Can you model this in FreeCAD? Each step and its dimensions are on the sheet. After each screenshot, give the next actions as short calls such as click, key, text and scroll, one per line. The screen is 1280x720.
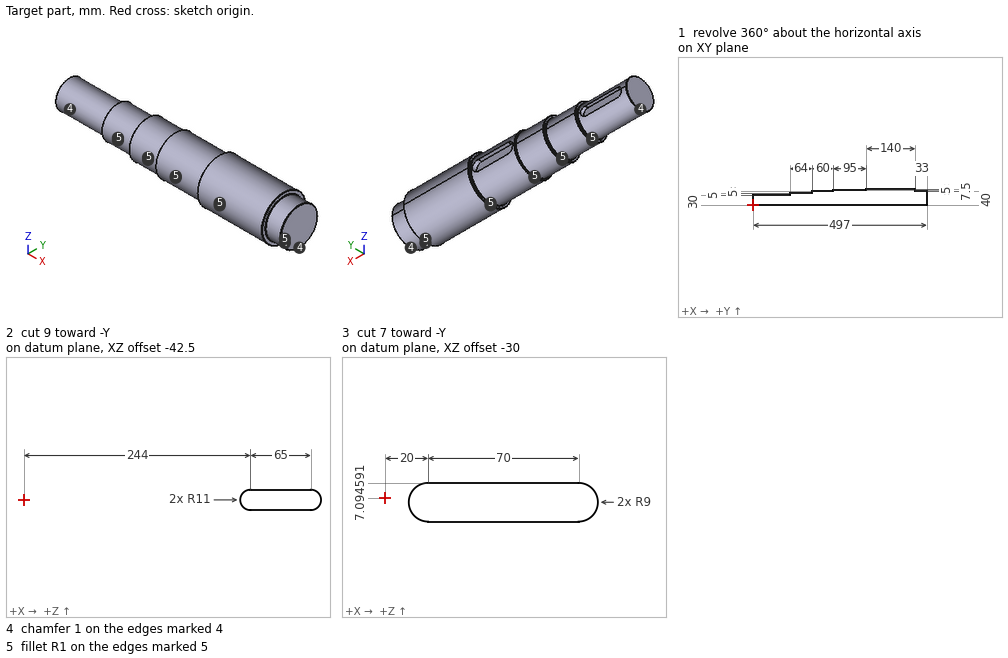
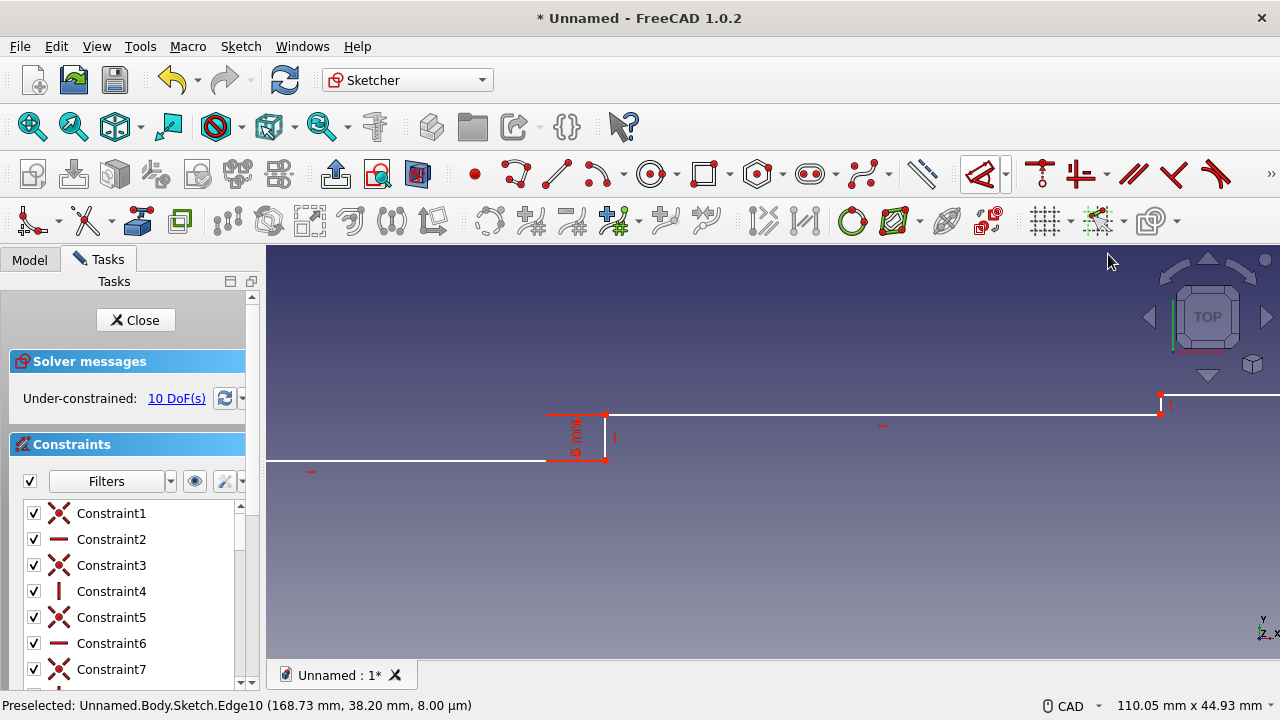
scroll(605, 435, down, 10)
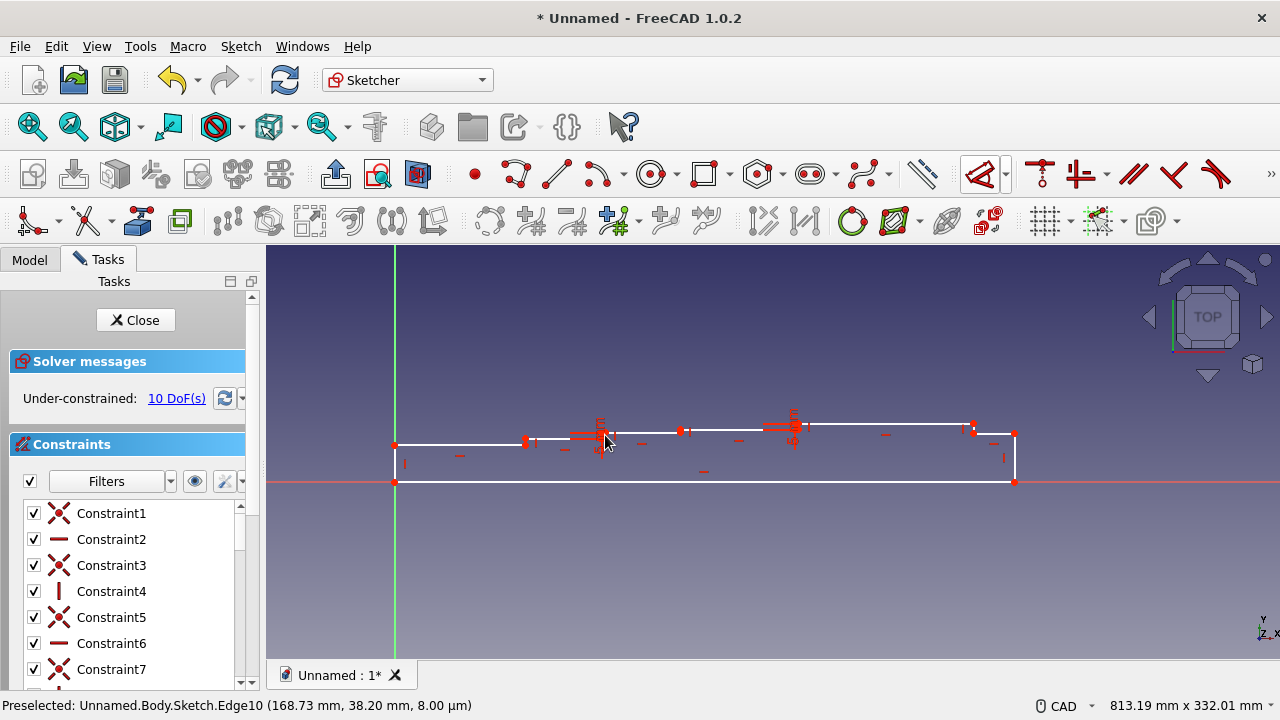
scroll(526, 441, up, 10)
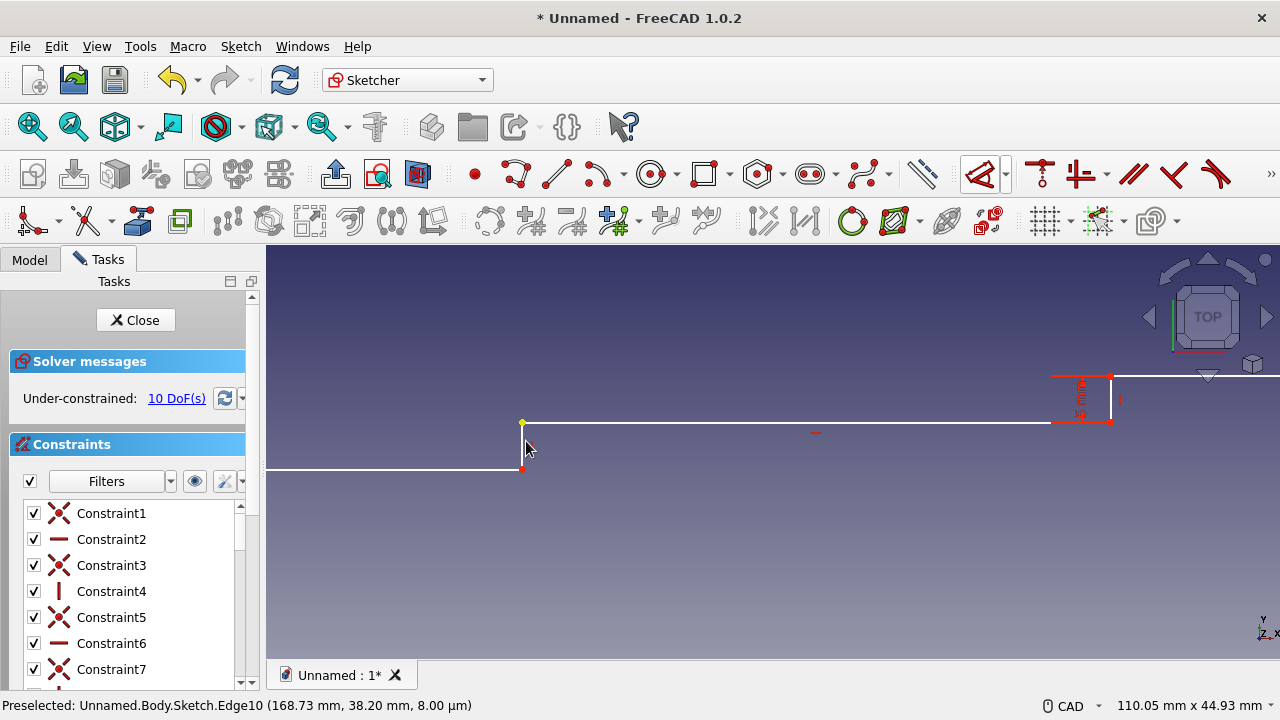
click(522, 437)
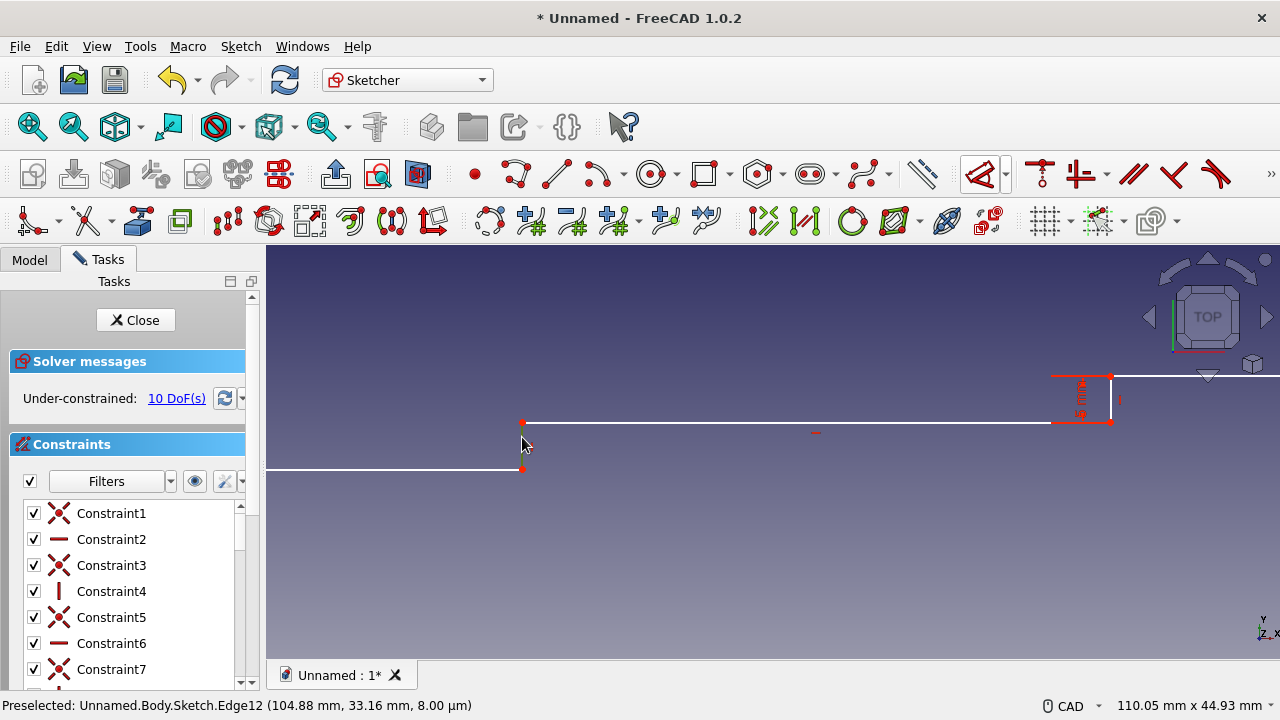
key(i)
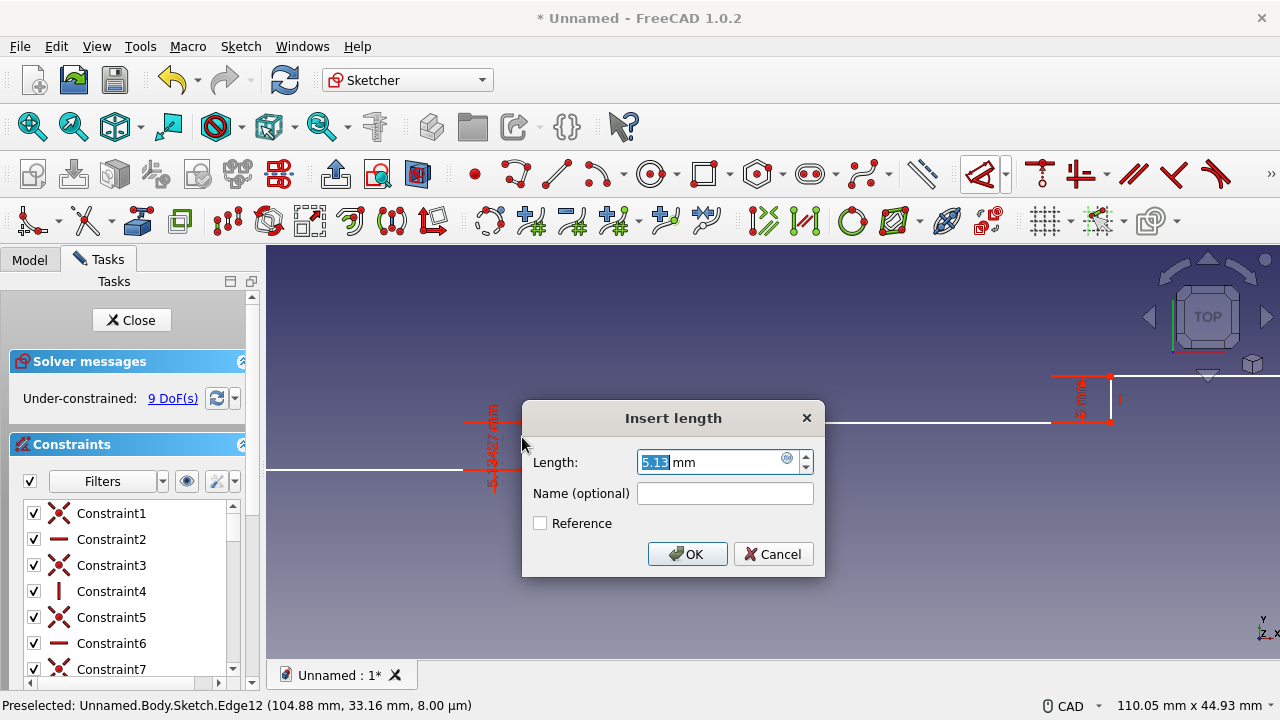
text(5)
key(Return)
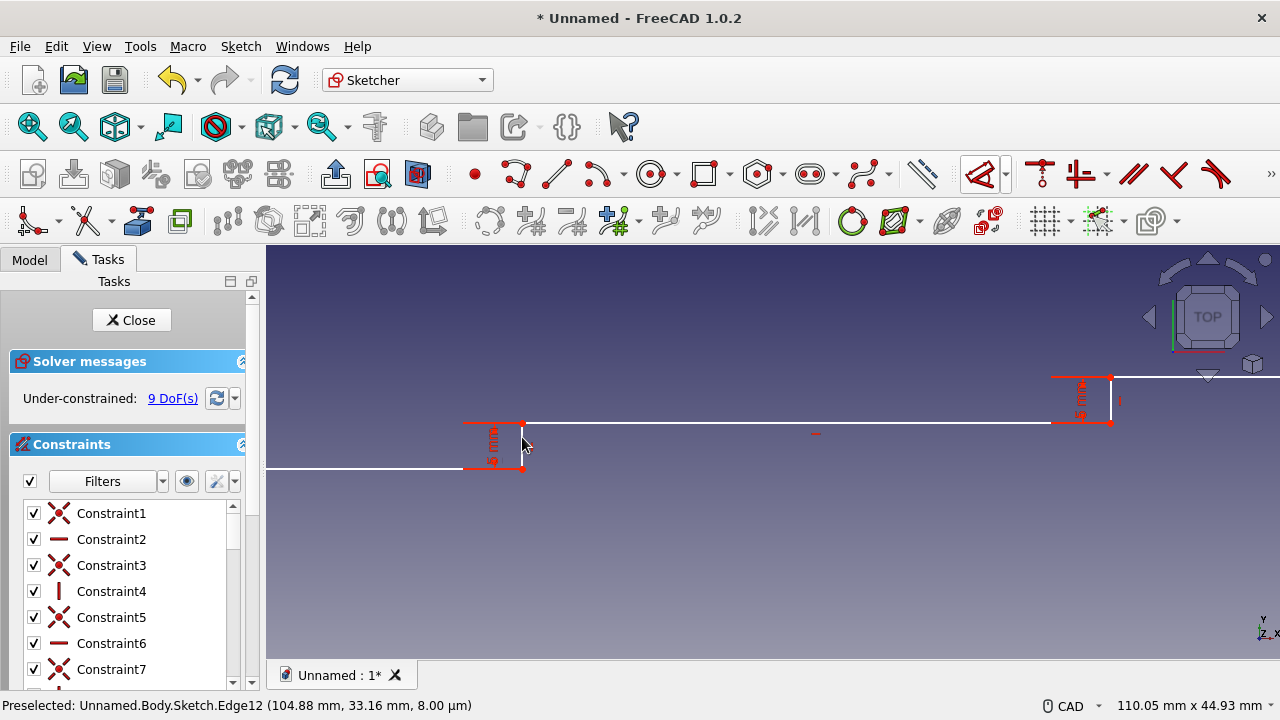
scroll(526, 441, down, 10)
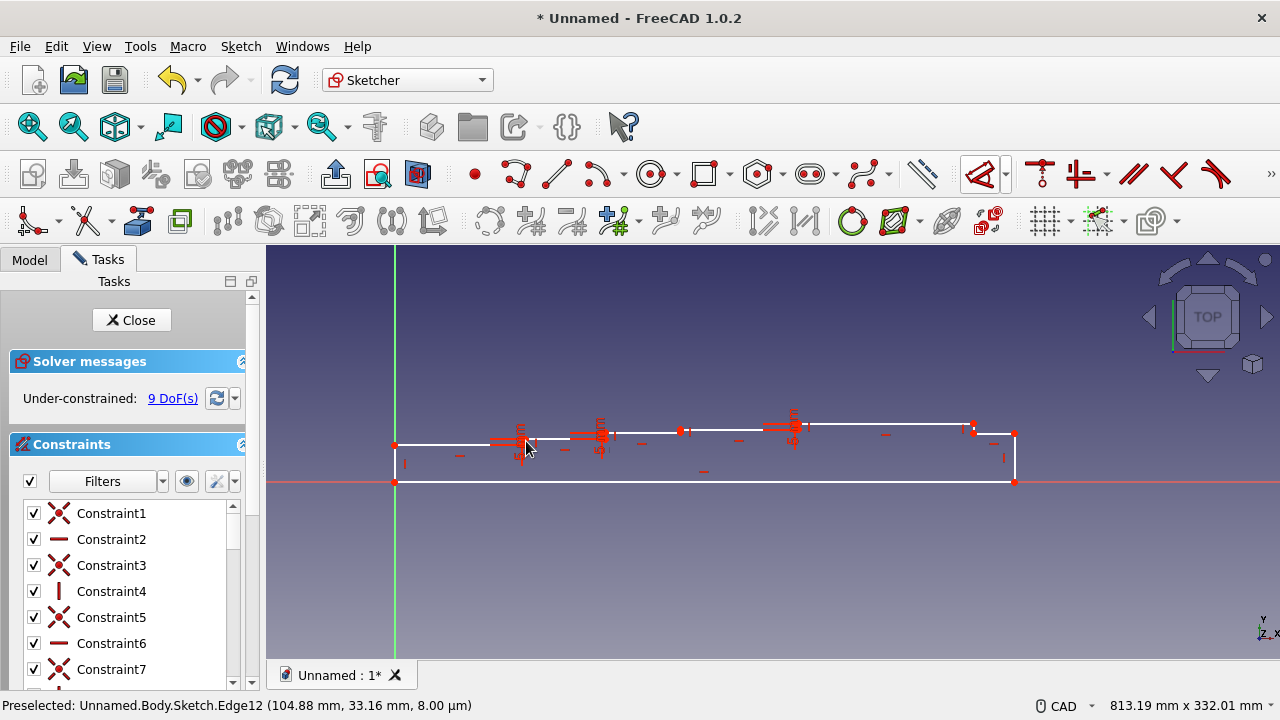
click(1015, 468)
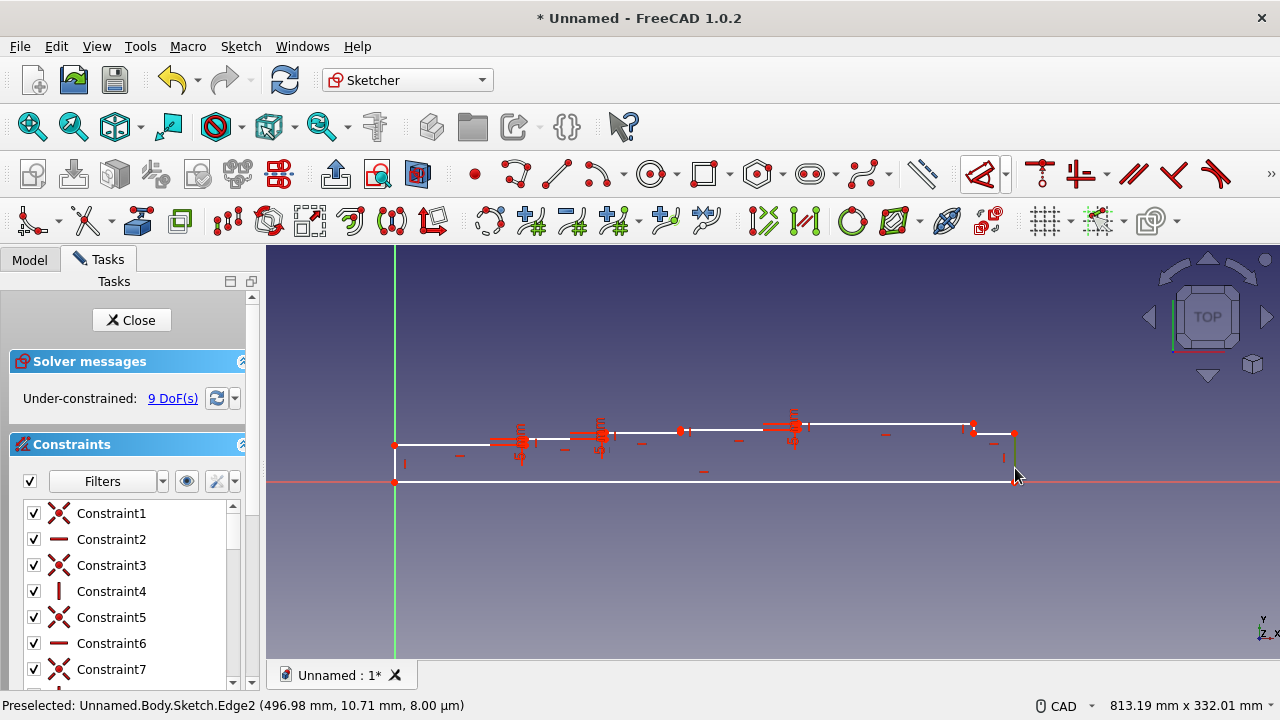
key(i)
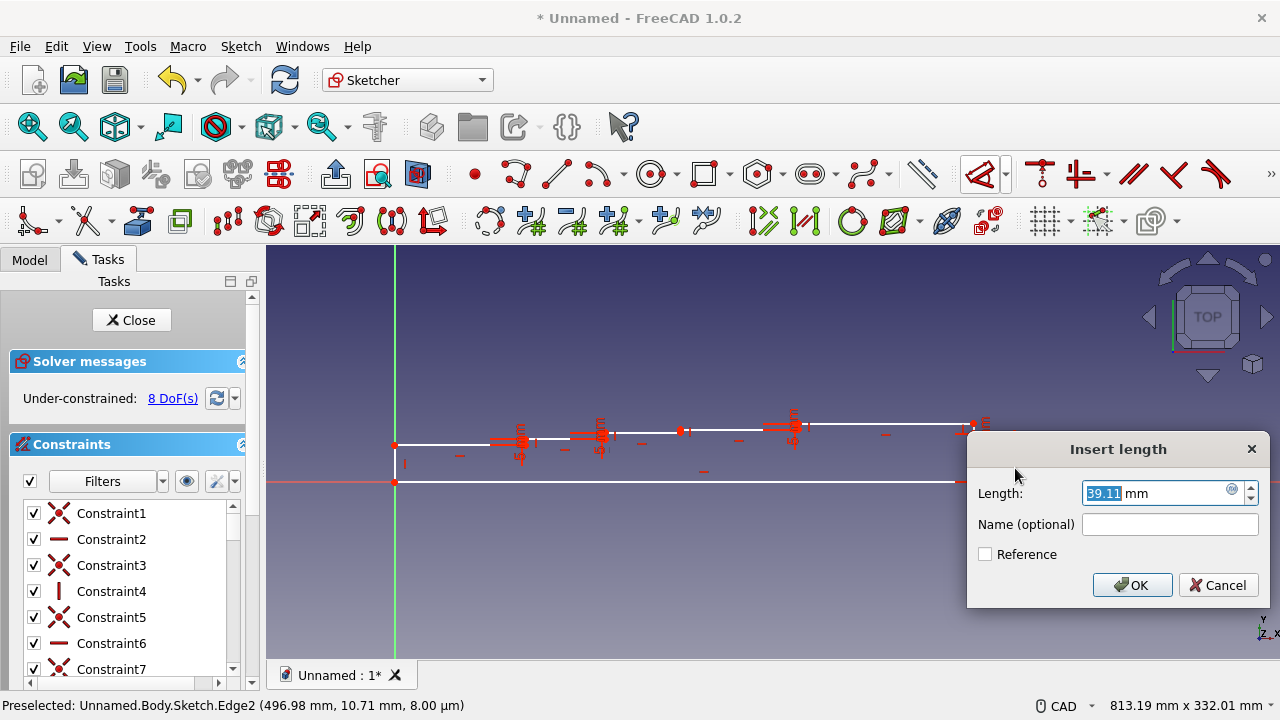
text(40)
key(Return)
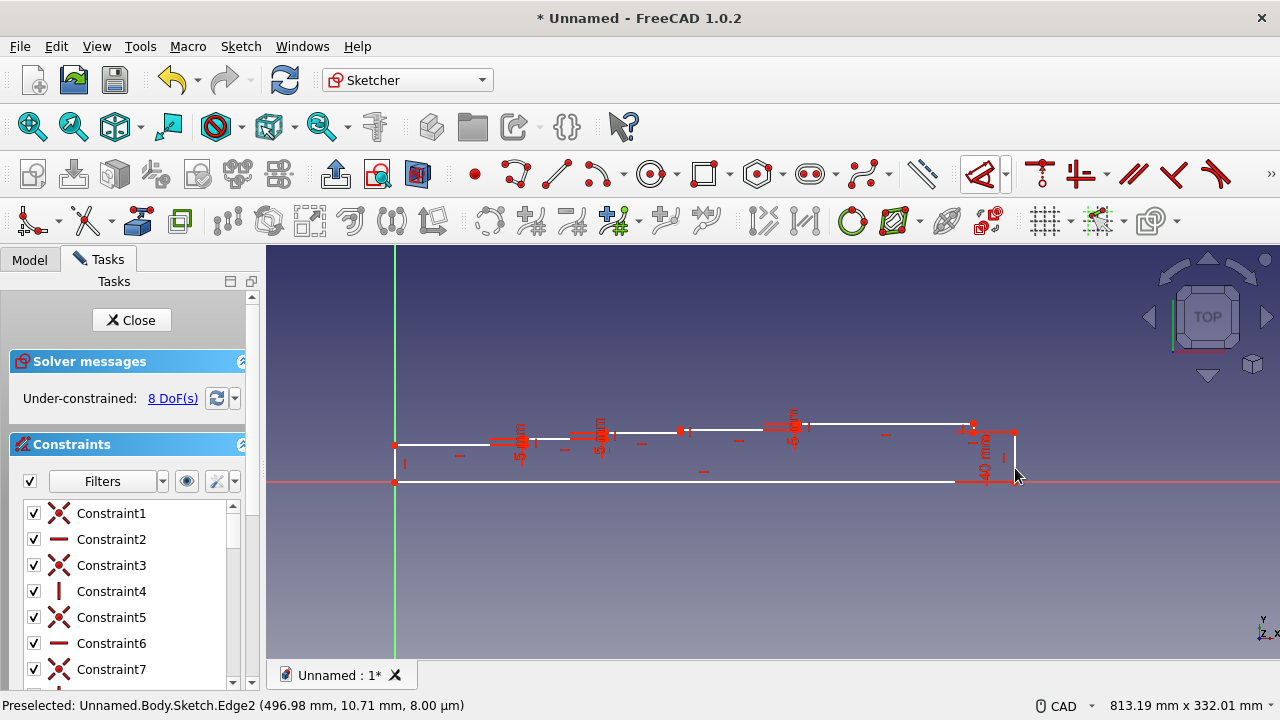
click(1002, 432)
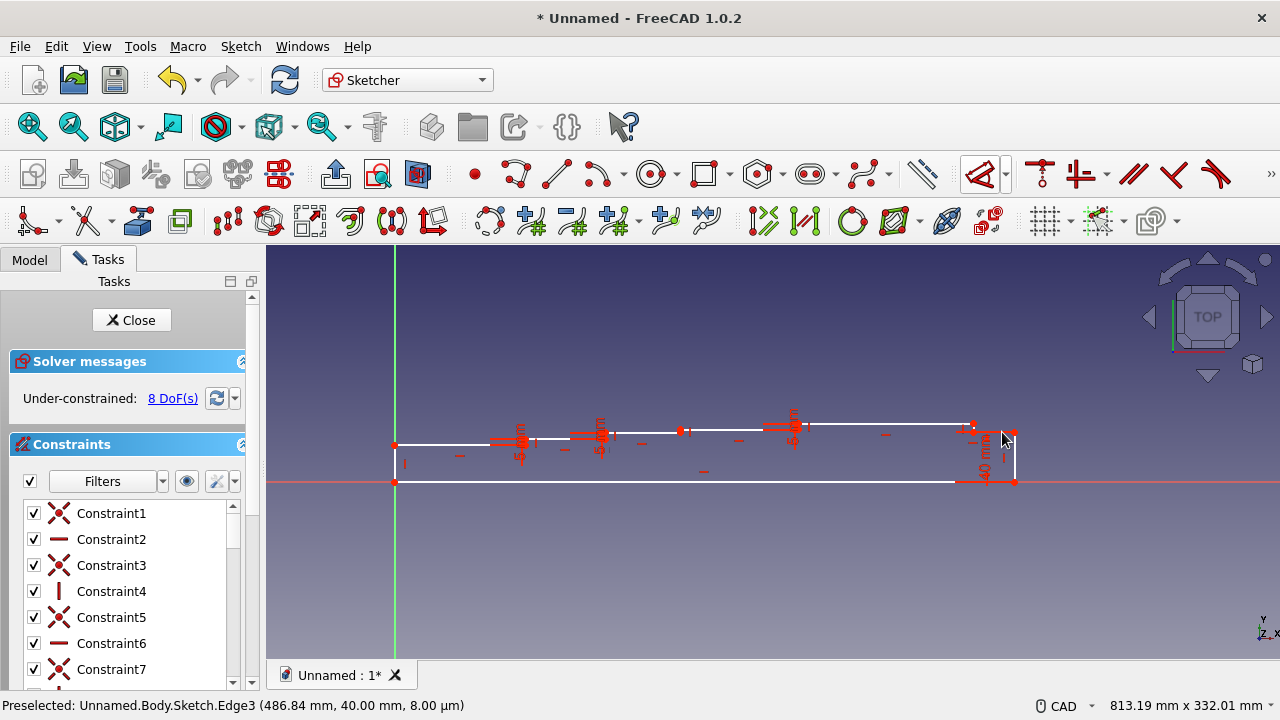
key(l)